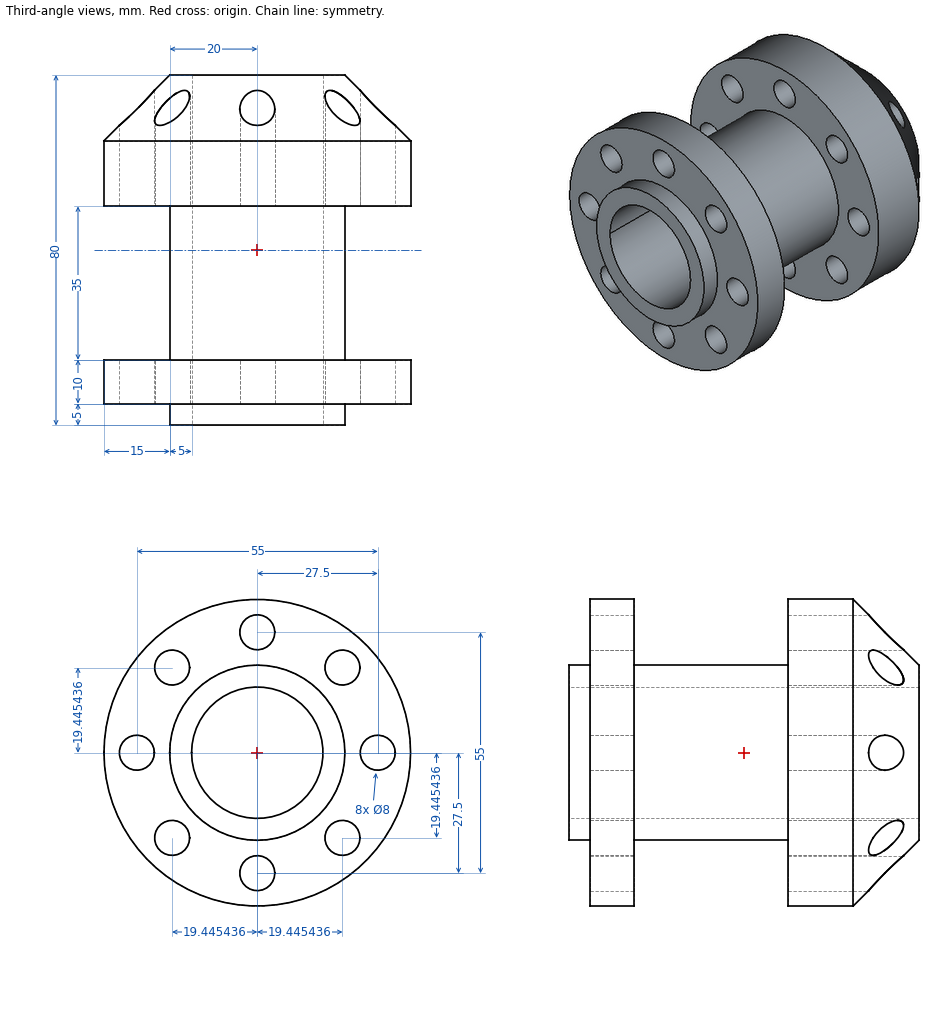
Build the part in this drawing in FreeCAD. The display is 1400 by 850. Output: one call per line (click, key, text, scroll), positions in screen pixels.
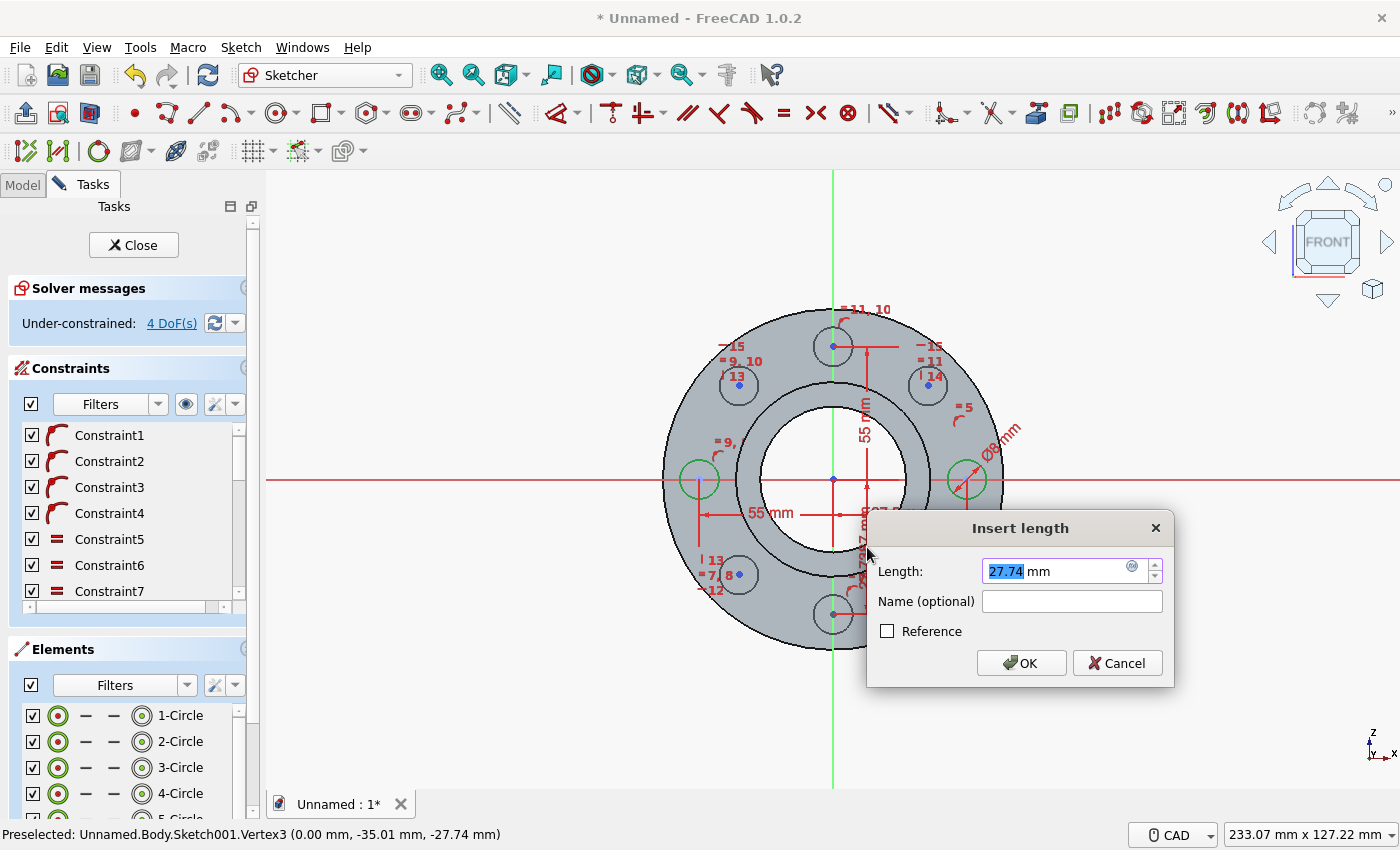
text(27.5)
key(Return)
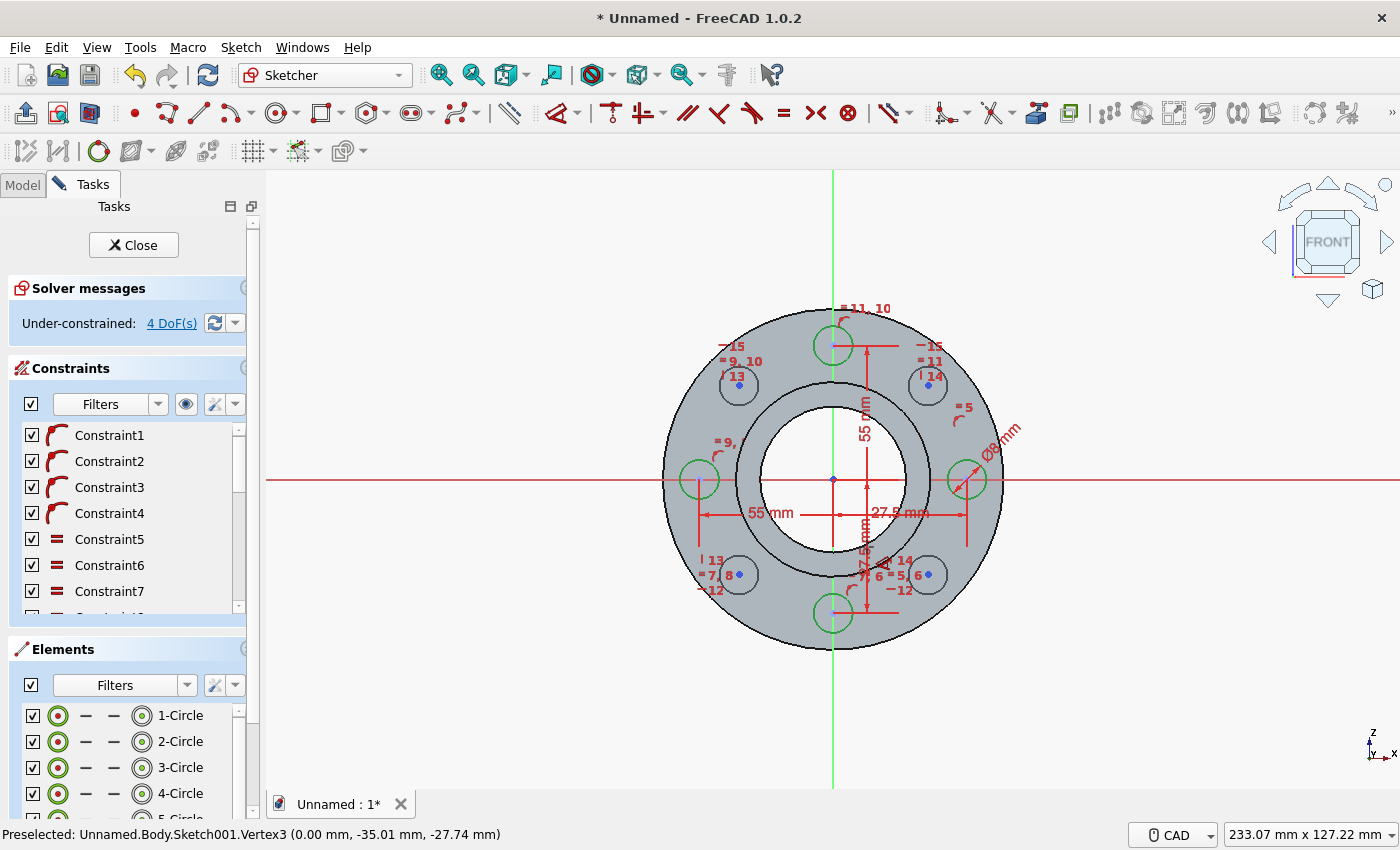
click(928, 575)
click(881, 609)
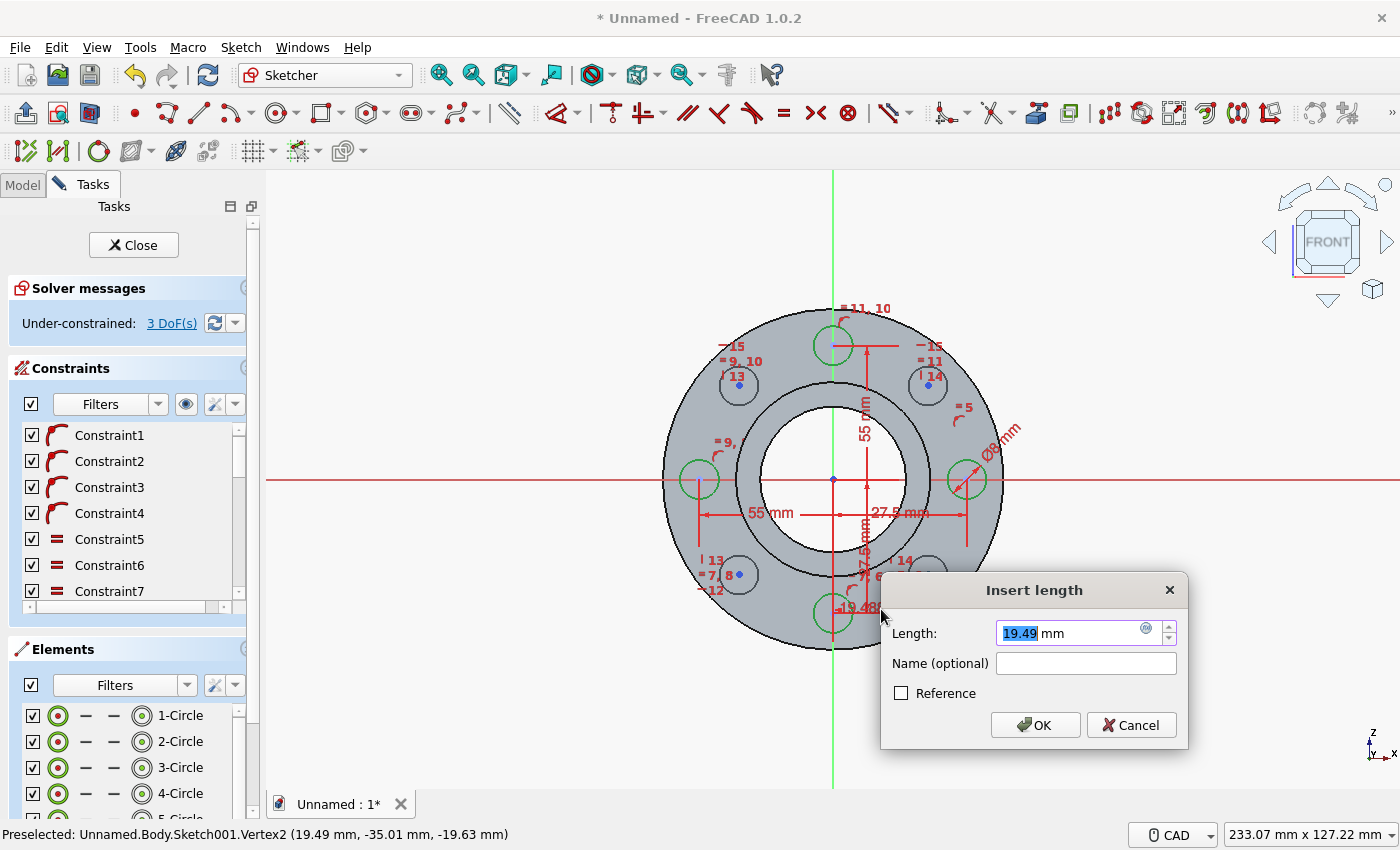
text(19.445436)
key(Return)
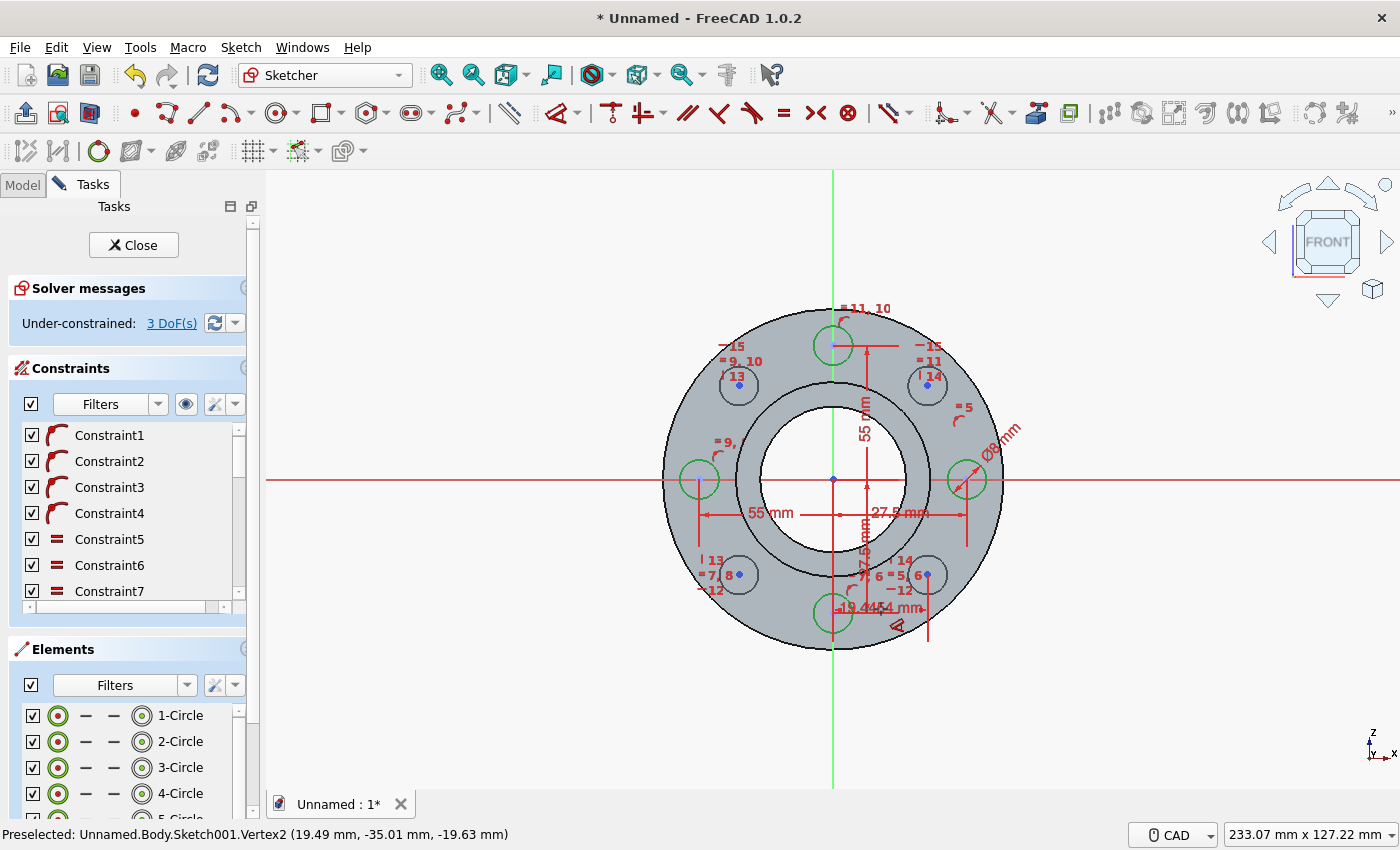
click(928, 575)
click(962, 549)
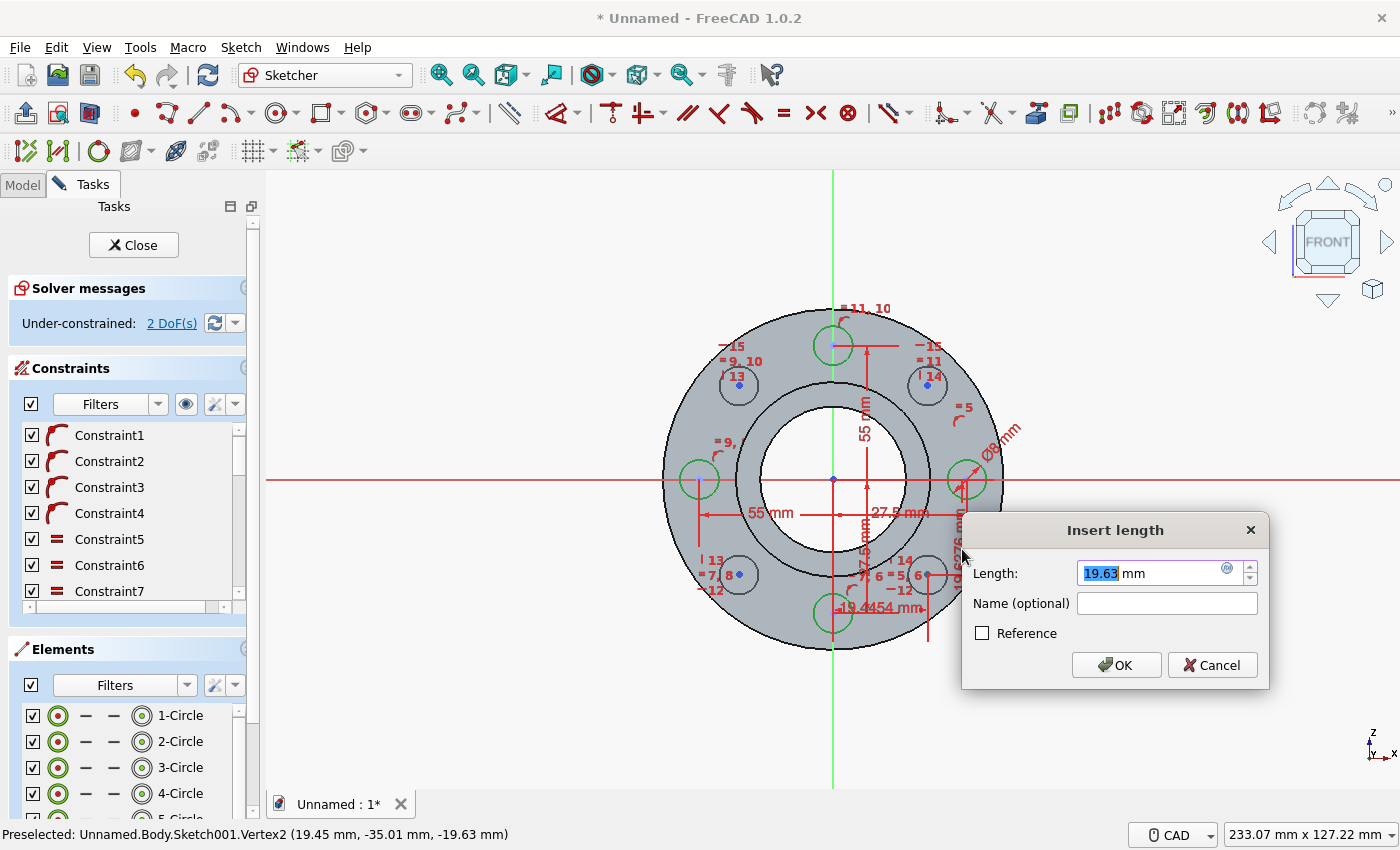
text(19.445436)
key(Return)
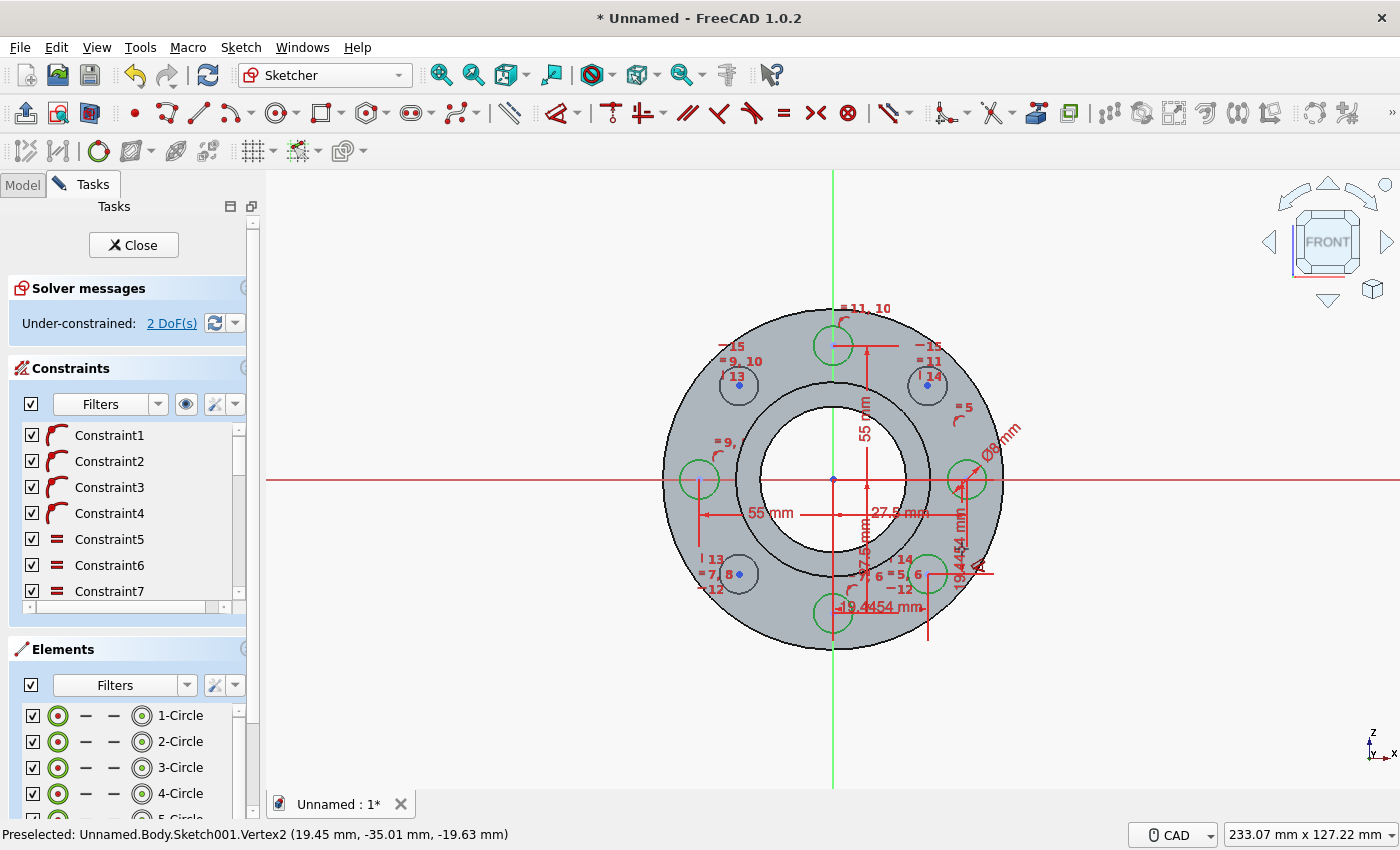
click(739, 574)
click(786, 608)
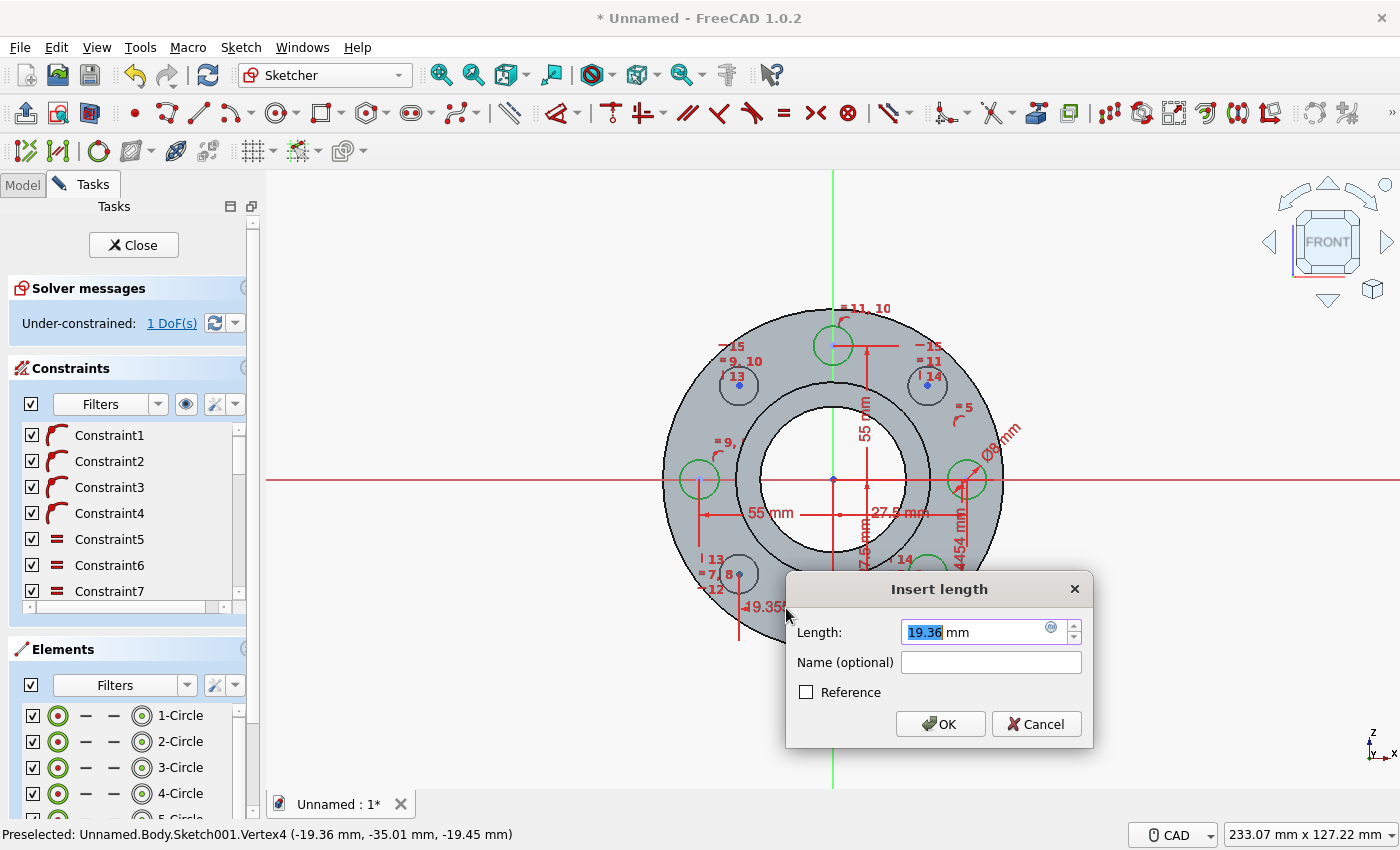
text(19.445436)
key(Return)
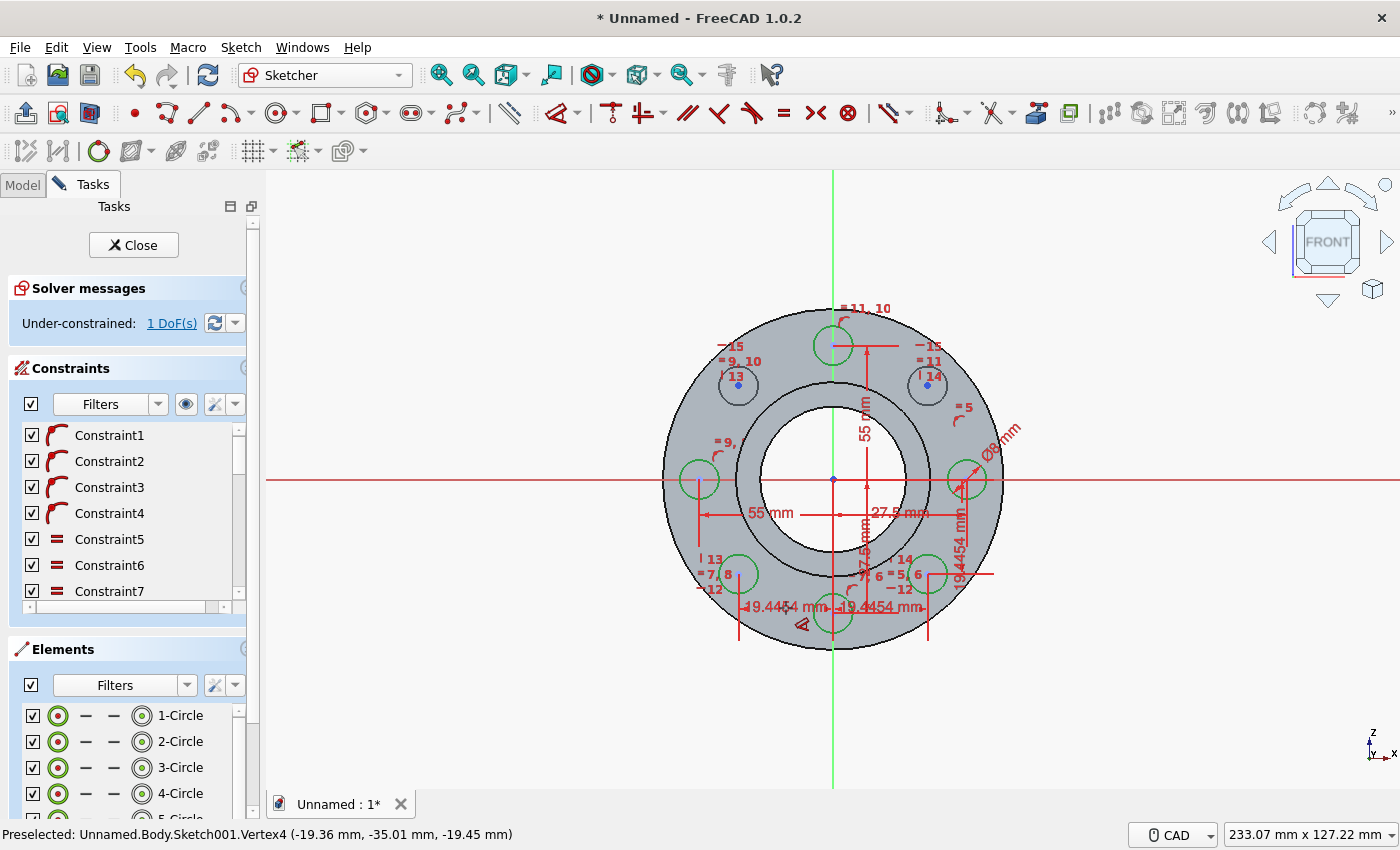
click(739, 386)
click(705, 433)